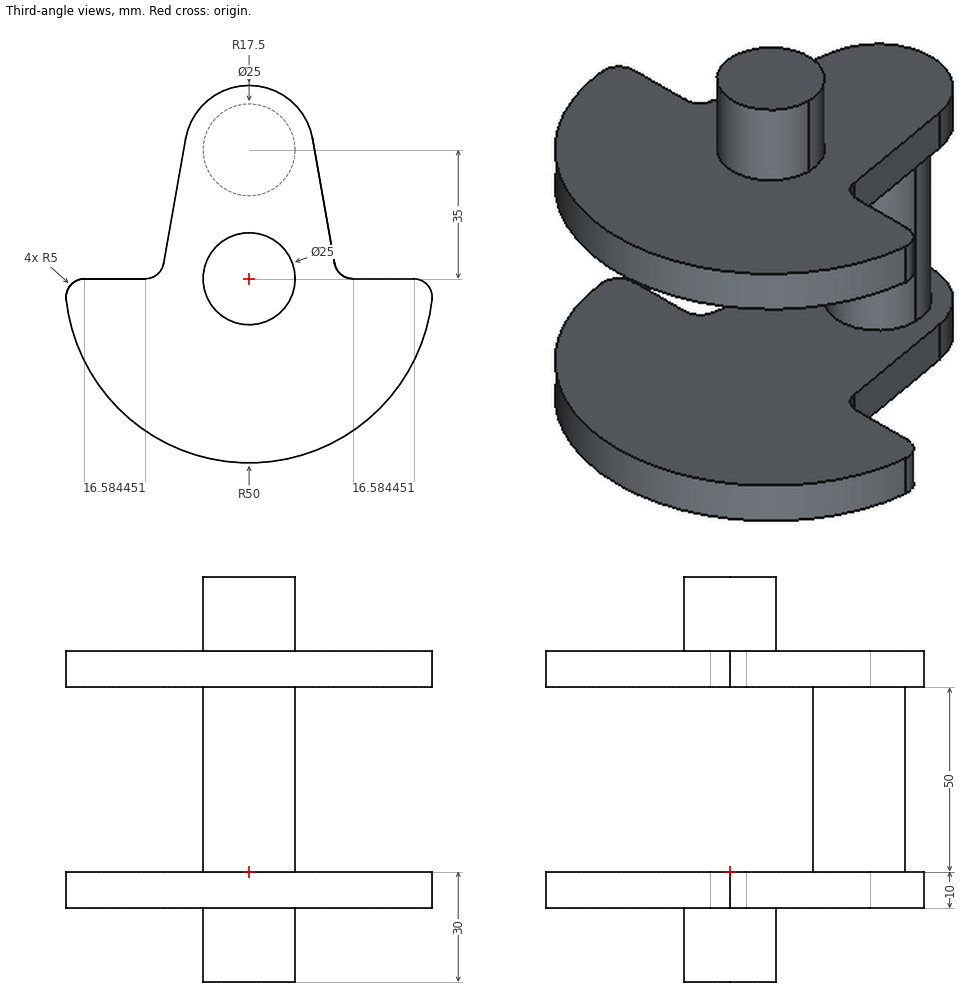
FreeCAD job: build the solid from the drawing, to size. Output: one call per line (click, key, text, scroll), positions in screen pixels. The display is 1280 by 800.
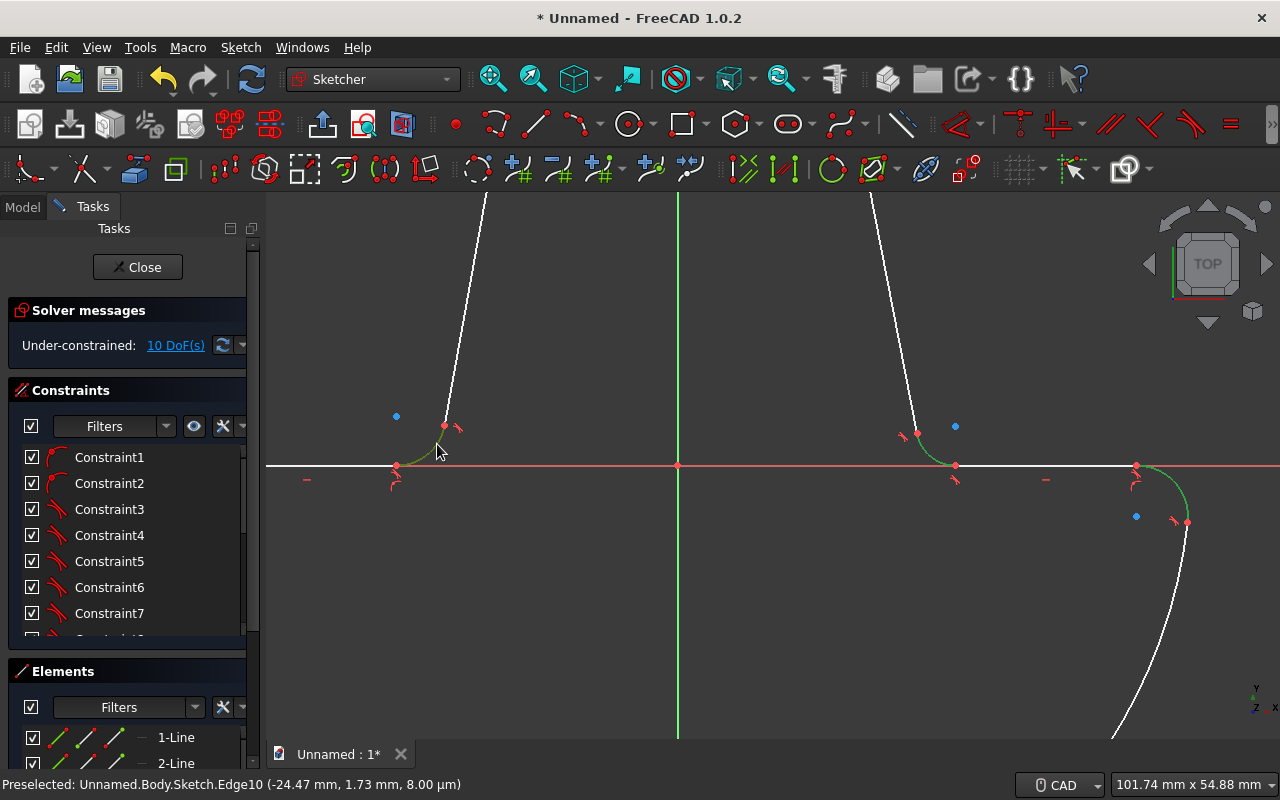
key(e)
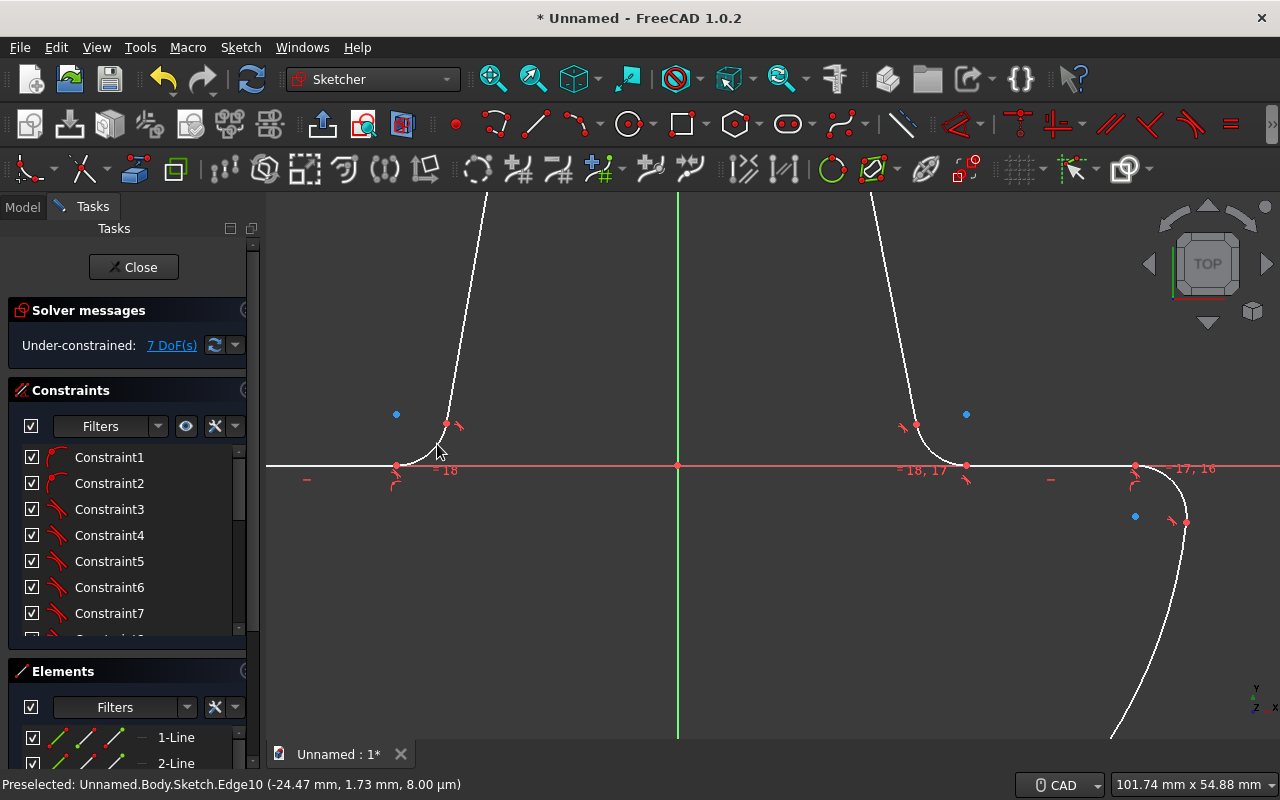
scroll(720, 473, down, 5)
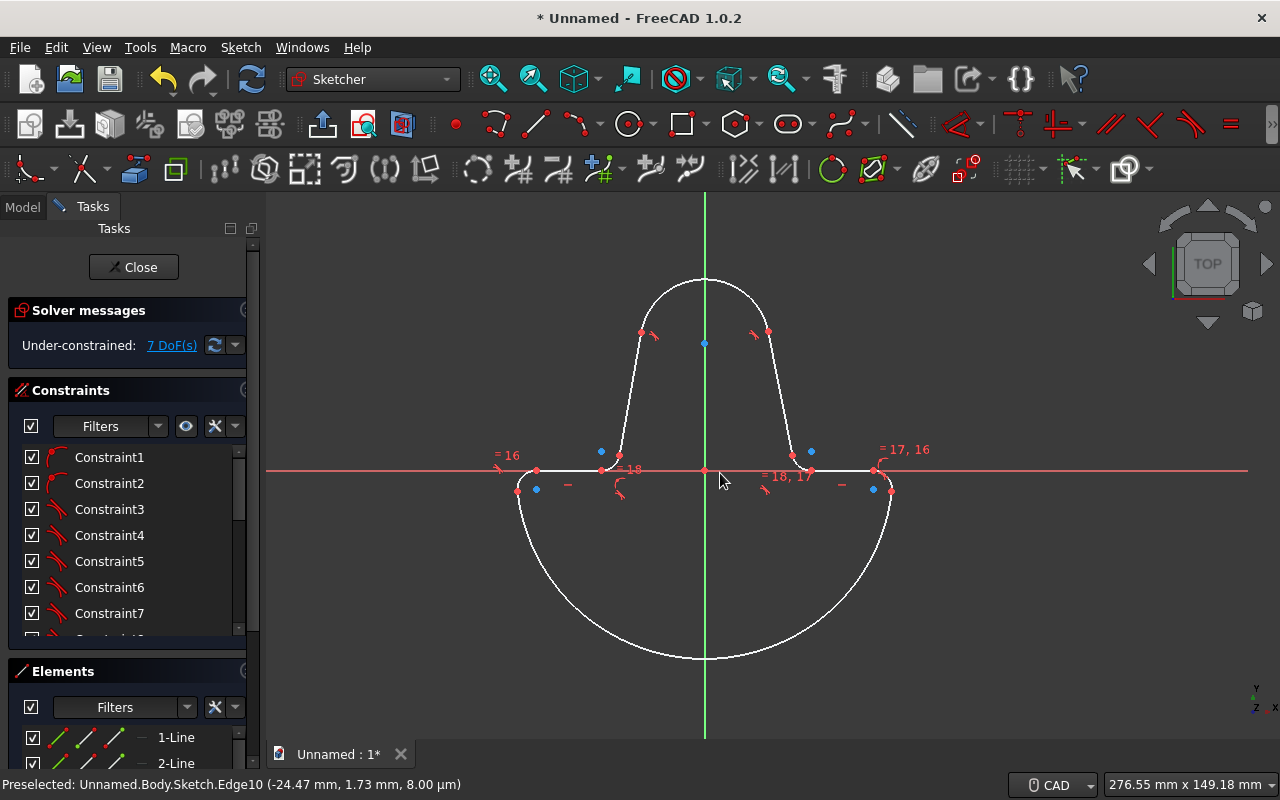
click(705, 344)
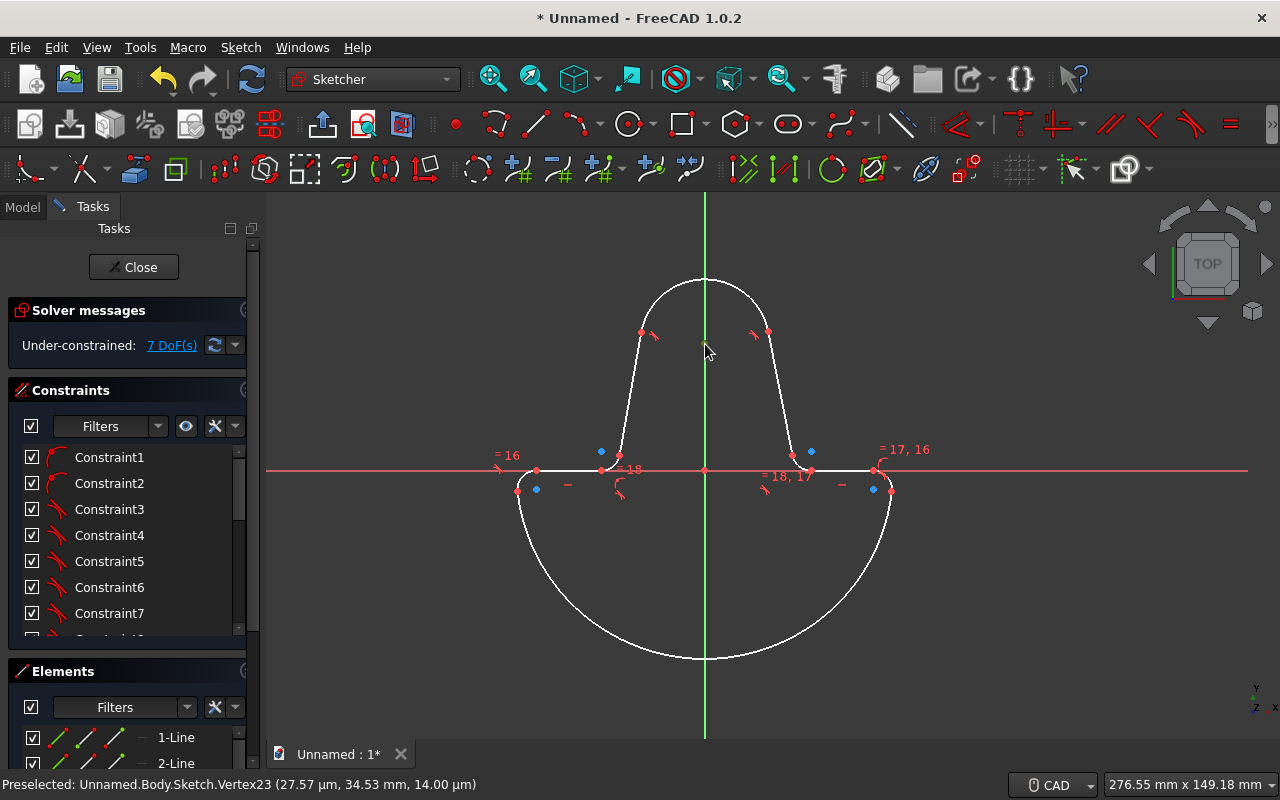
click(705, 606)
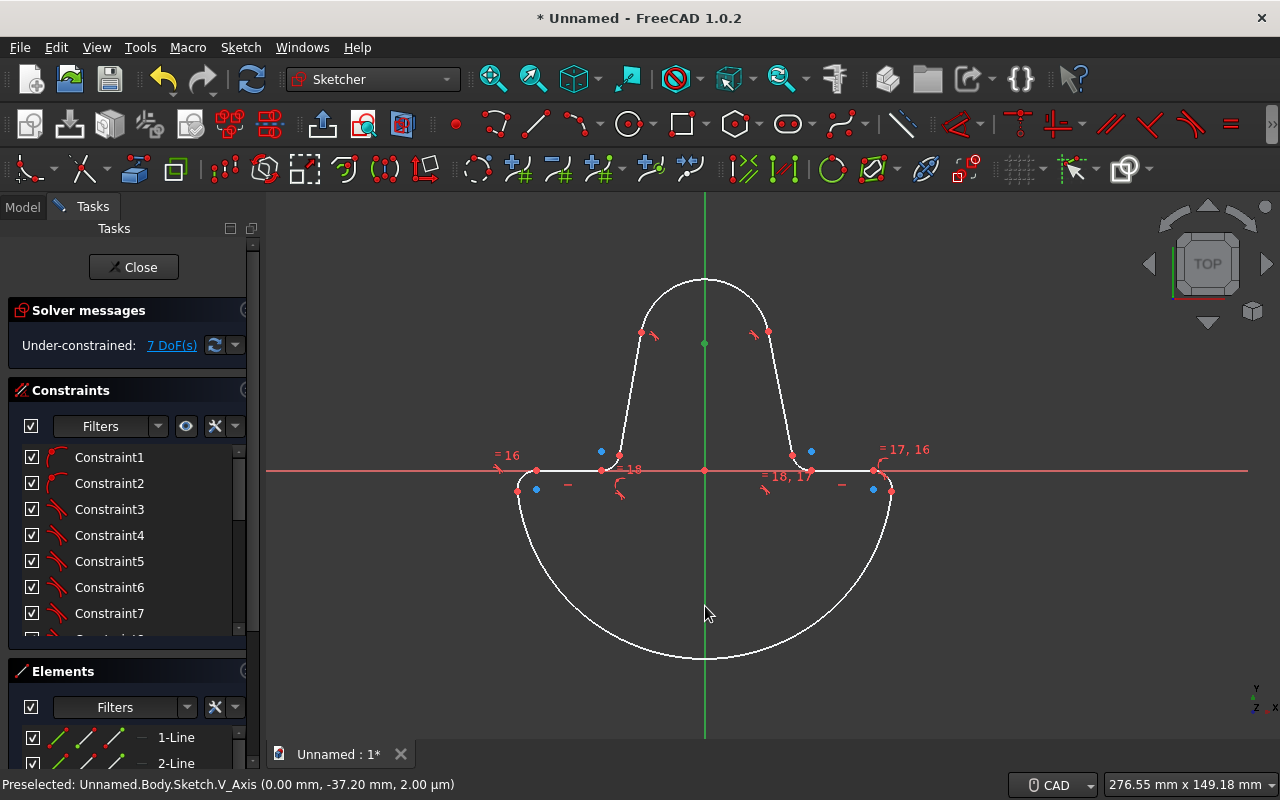
key(c)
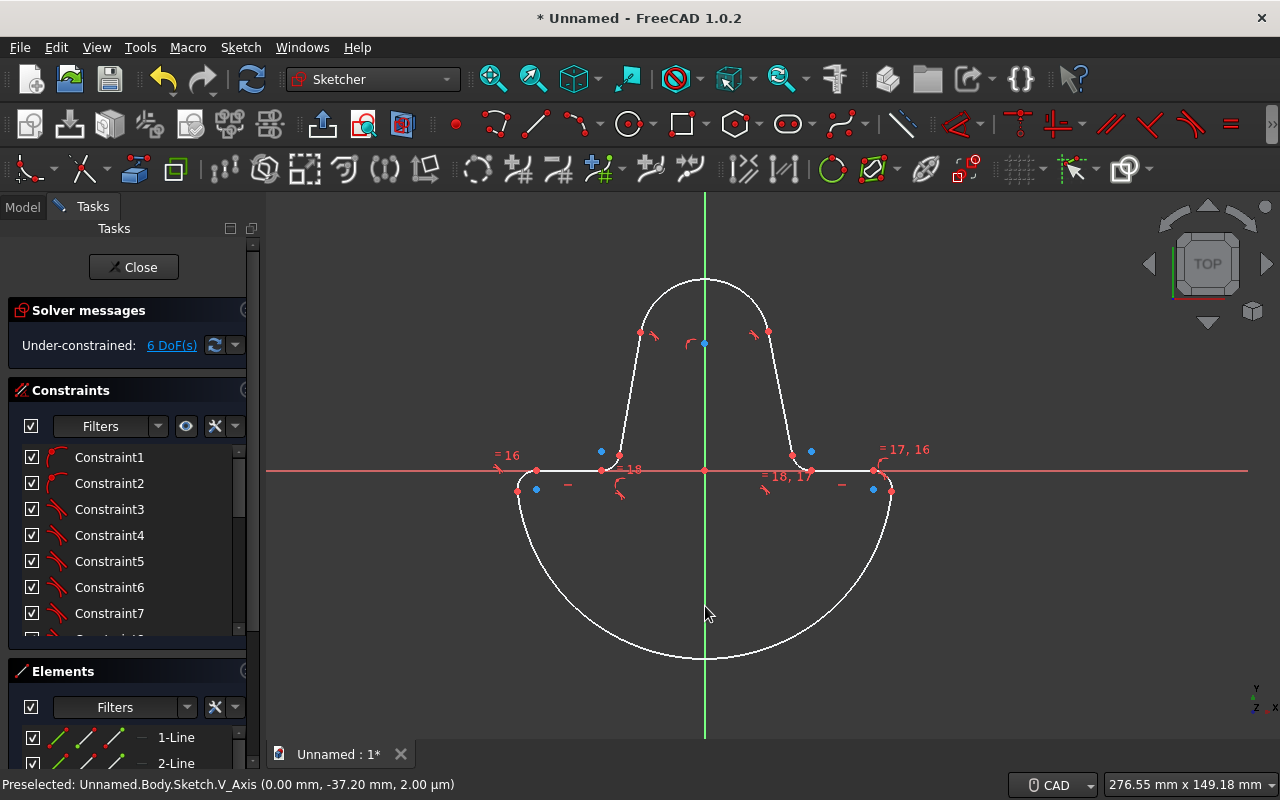
key(d)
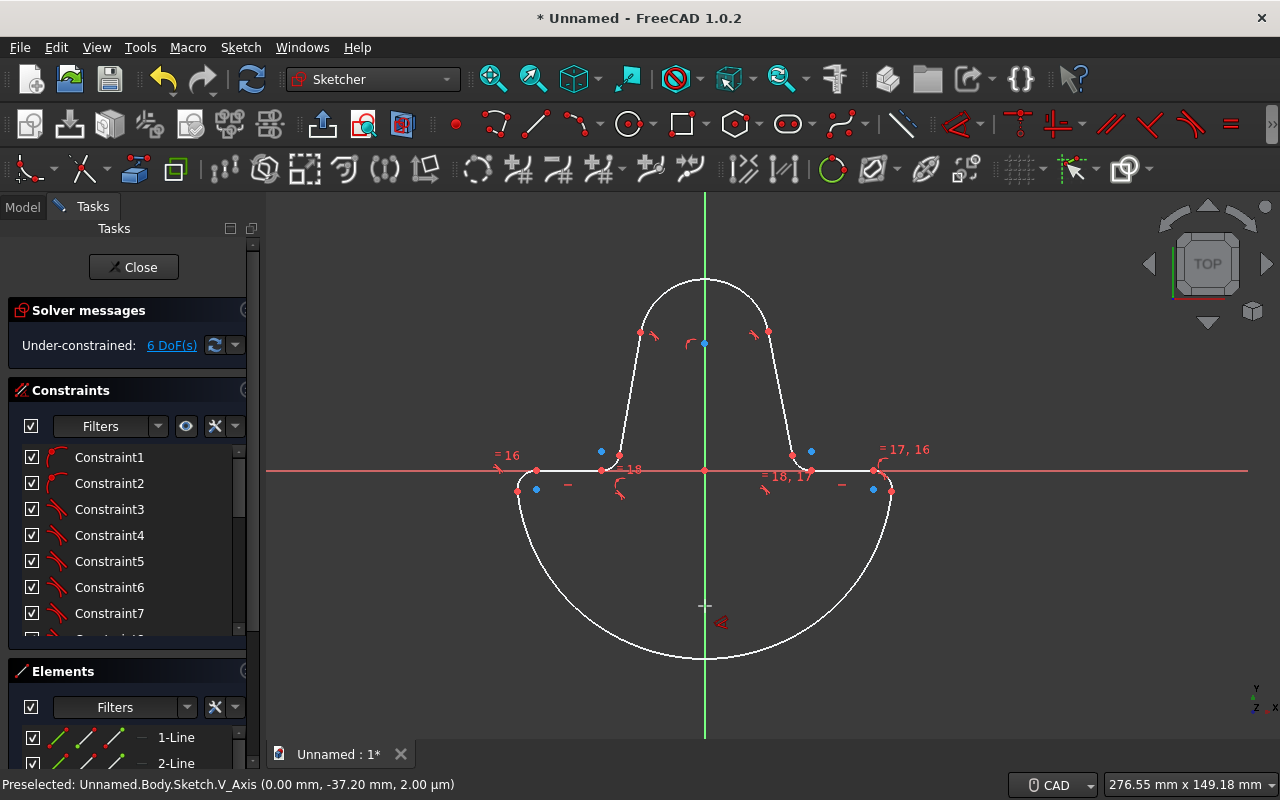
scroll(527, 473, up, 4)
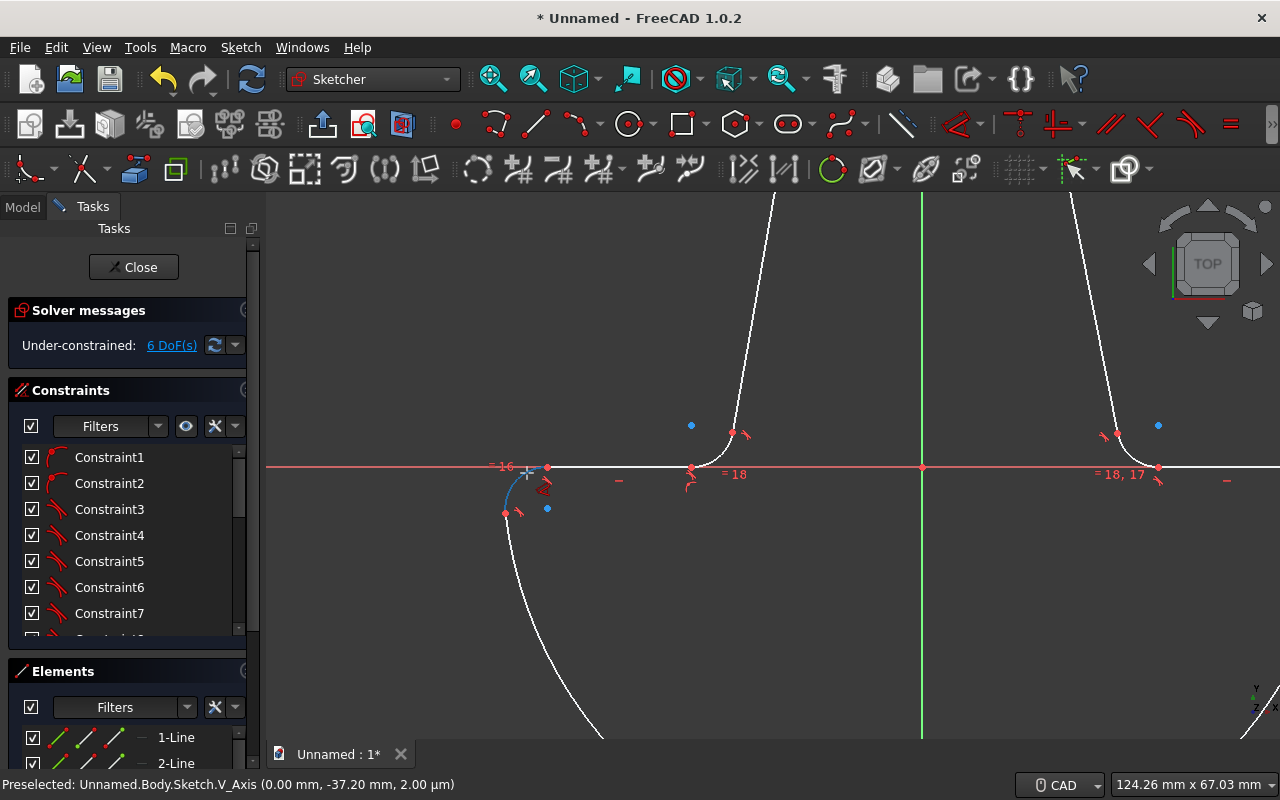
click(527, 472)
click(512, 444)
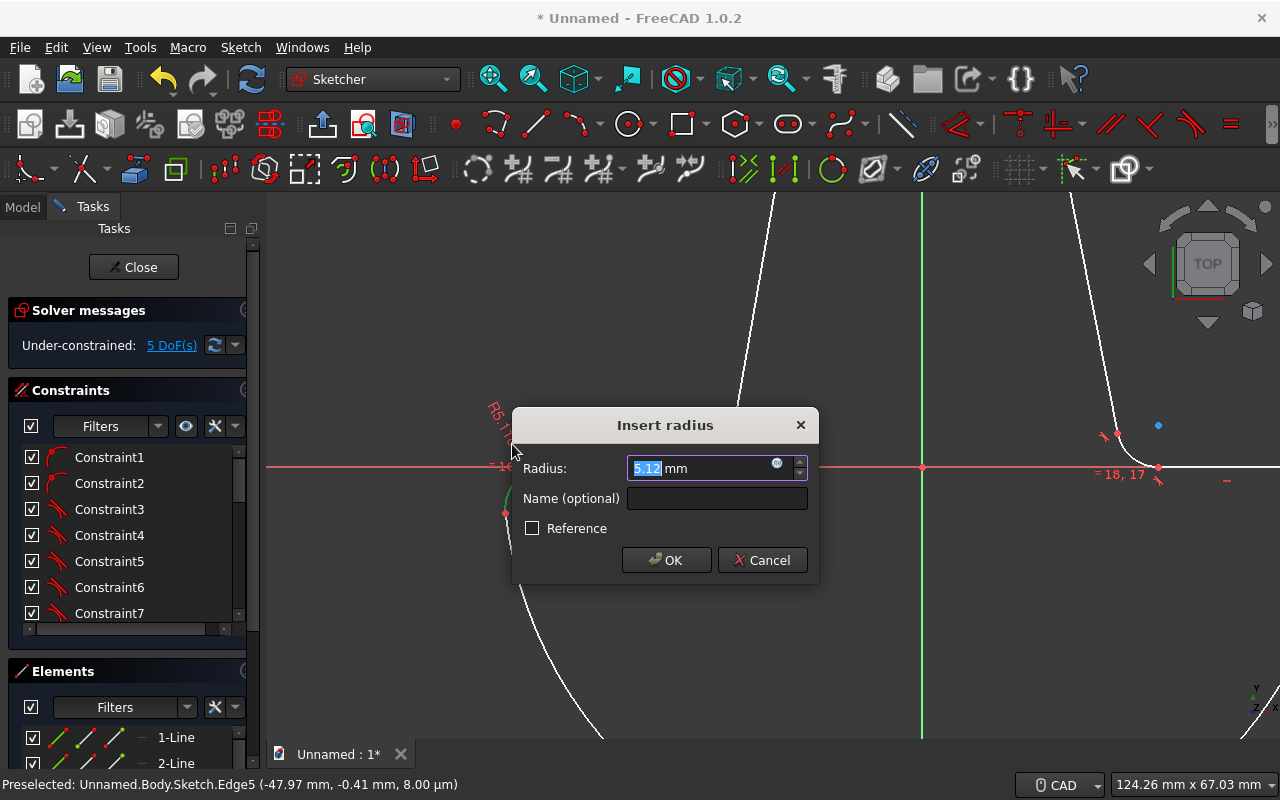
text(5)
key(Return)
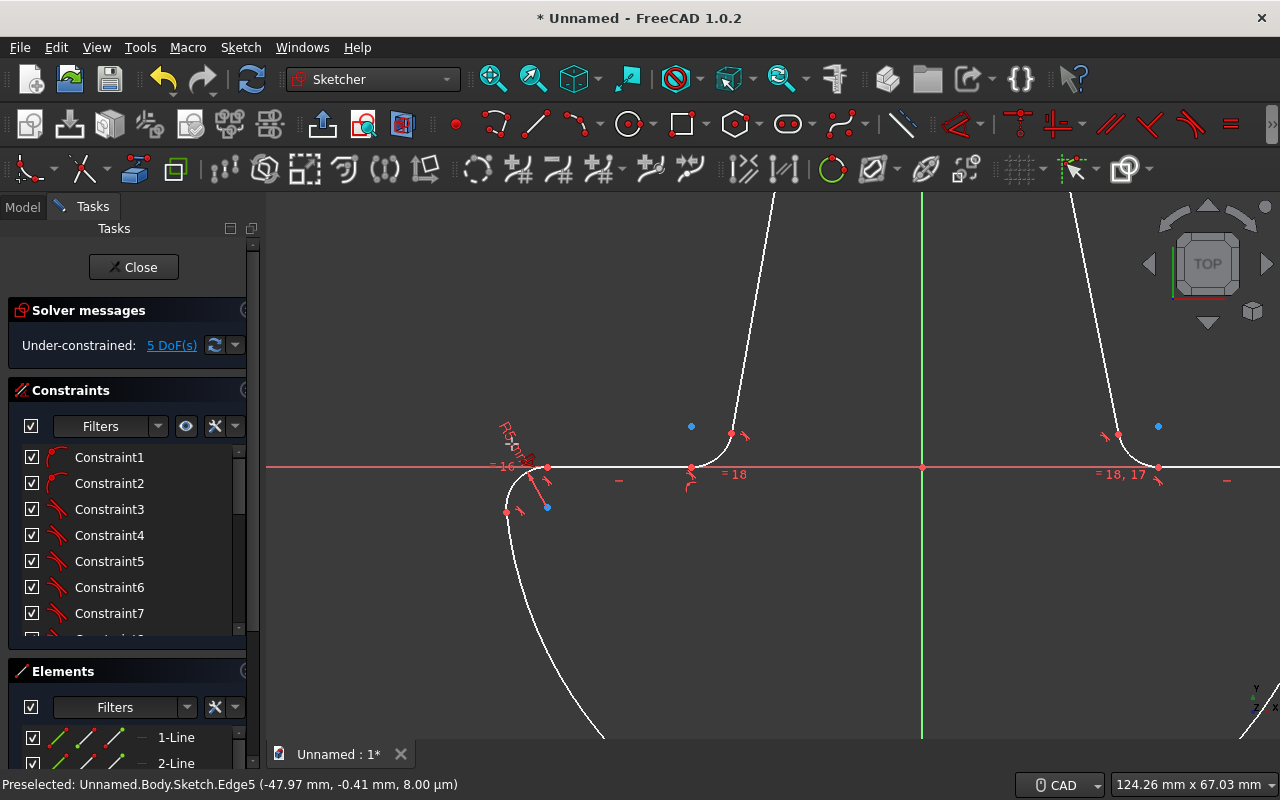
scroll(527, 473, down, 4)